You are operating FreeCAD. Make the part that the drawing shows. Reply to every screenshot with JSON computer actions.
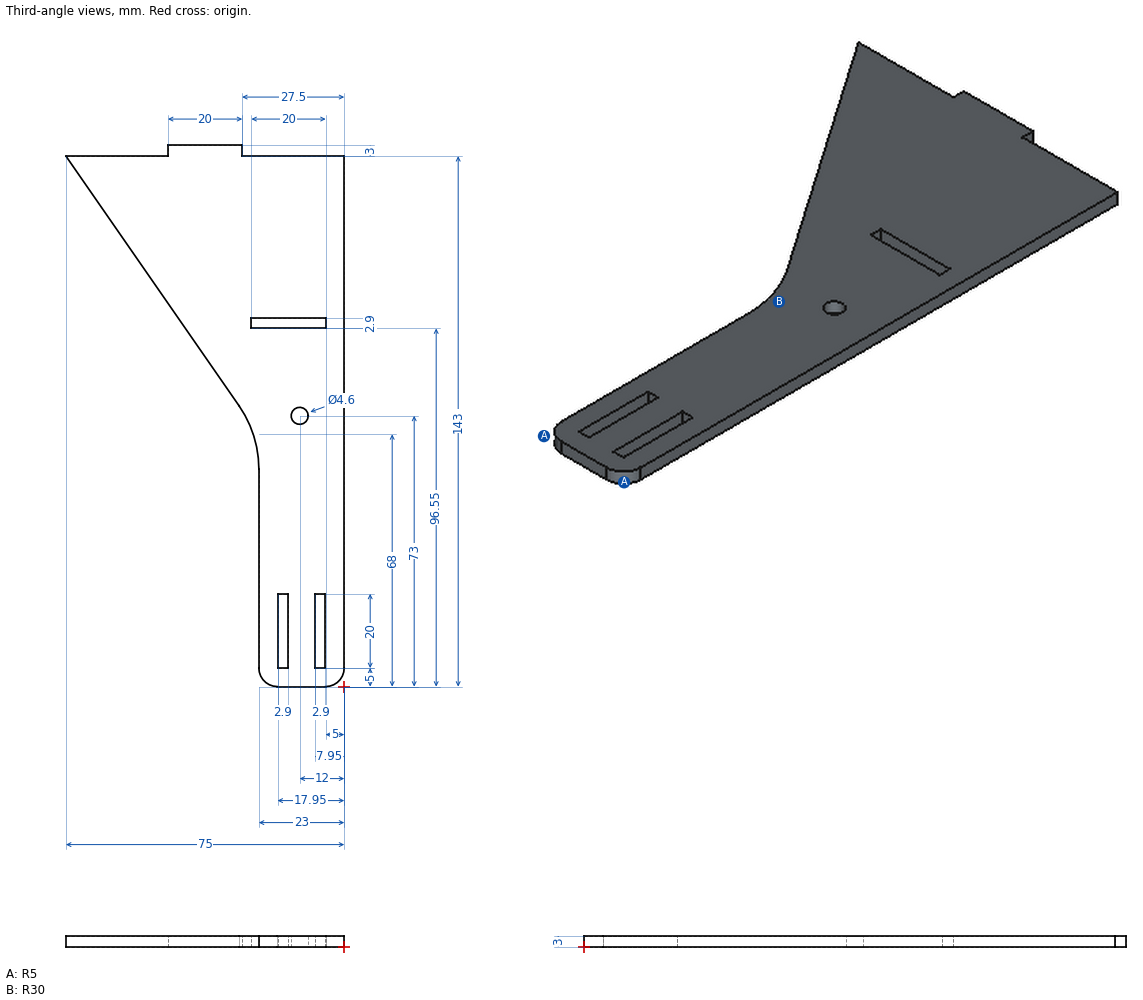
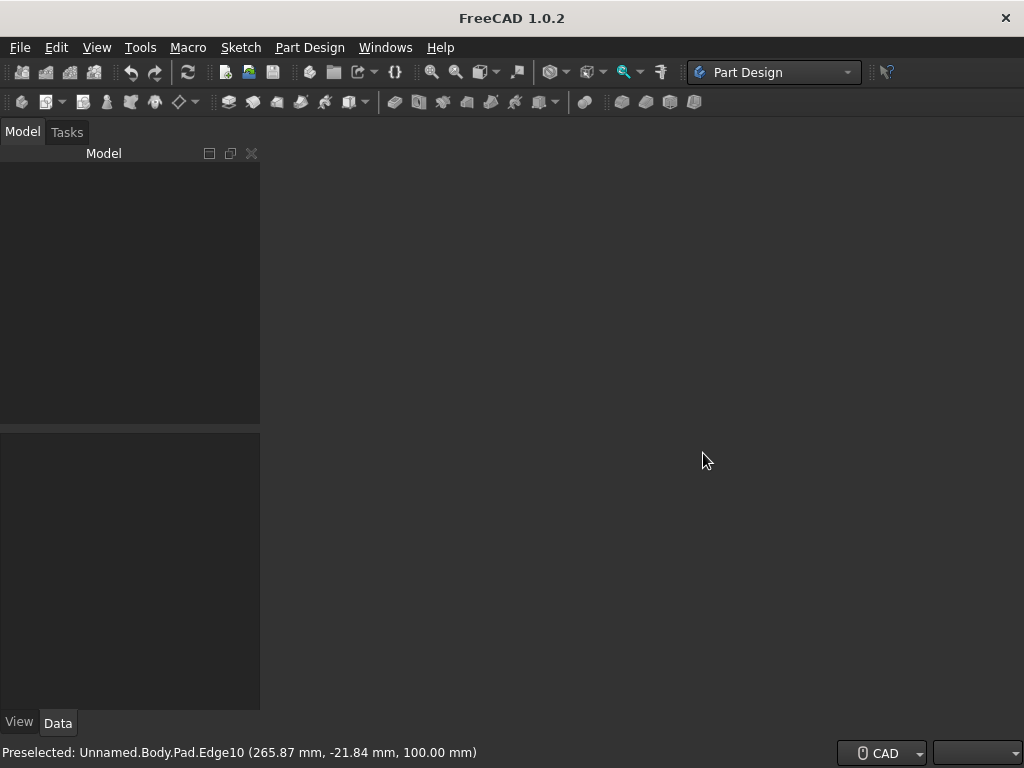
{"action": "left_click", "coordinate": [226, 72]}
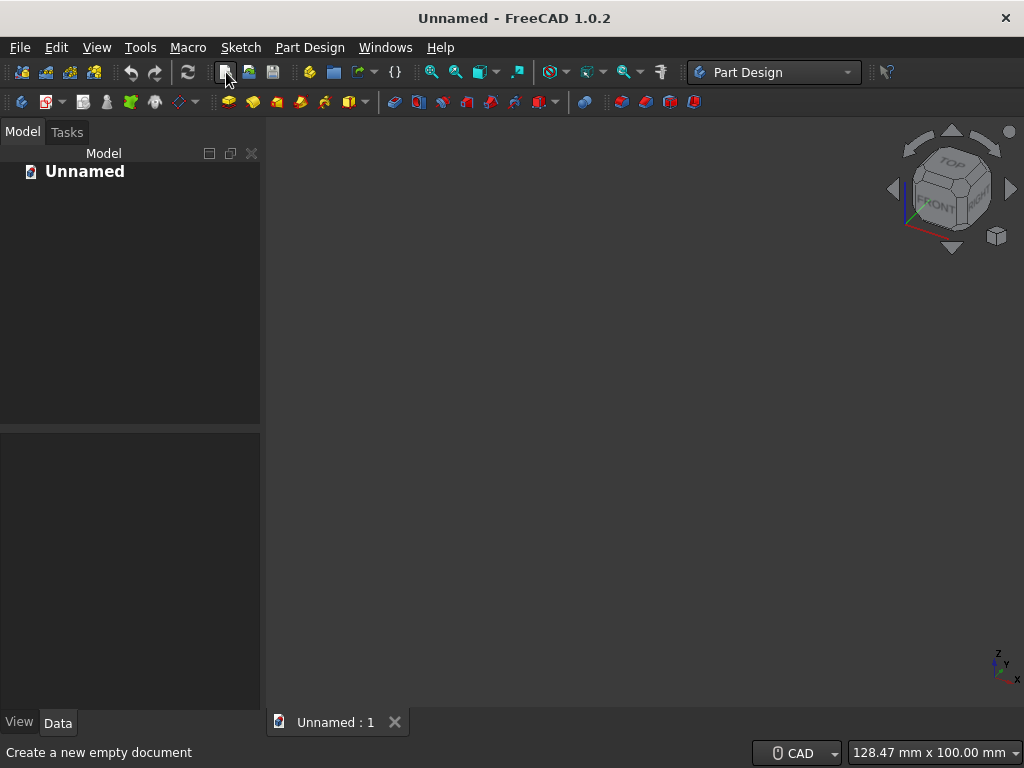
{"action": "left_click", "coordinate": [46, 102]}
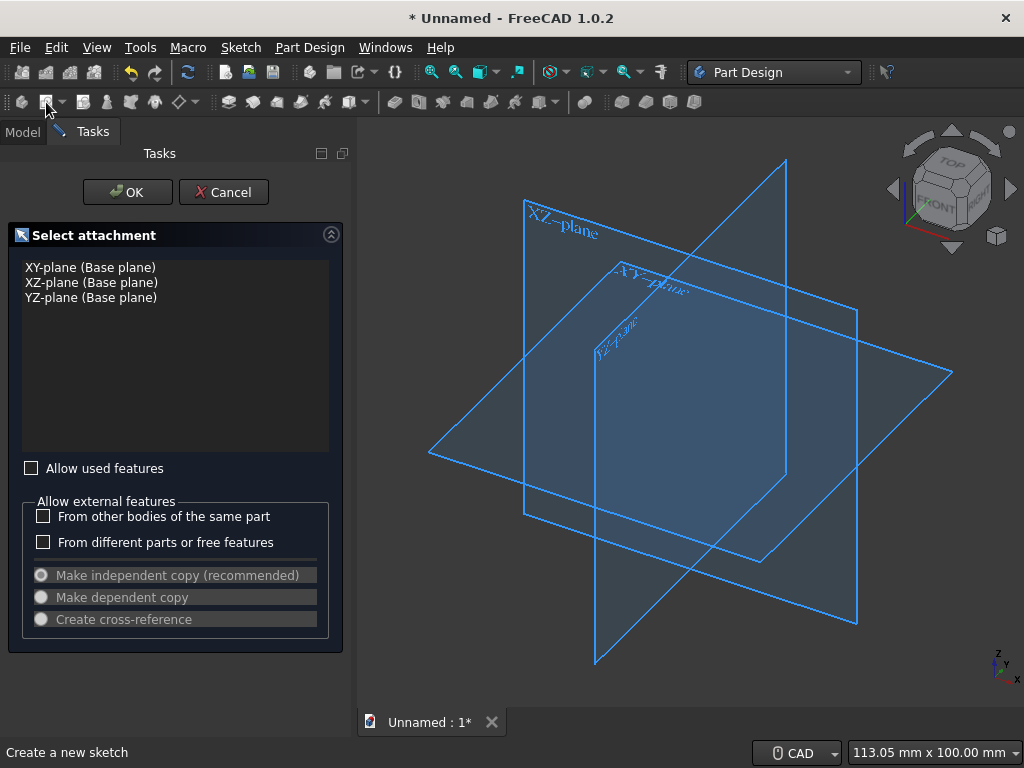
{"action": "left_click", "coordinate": [82, 268]}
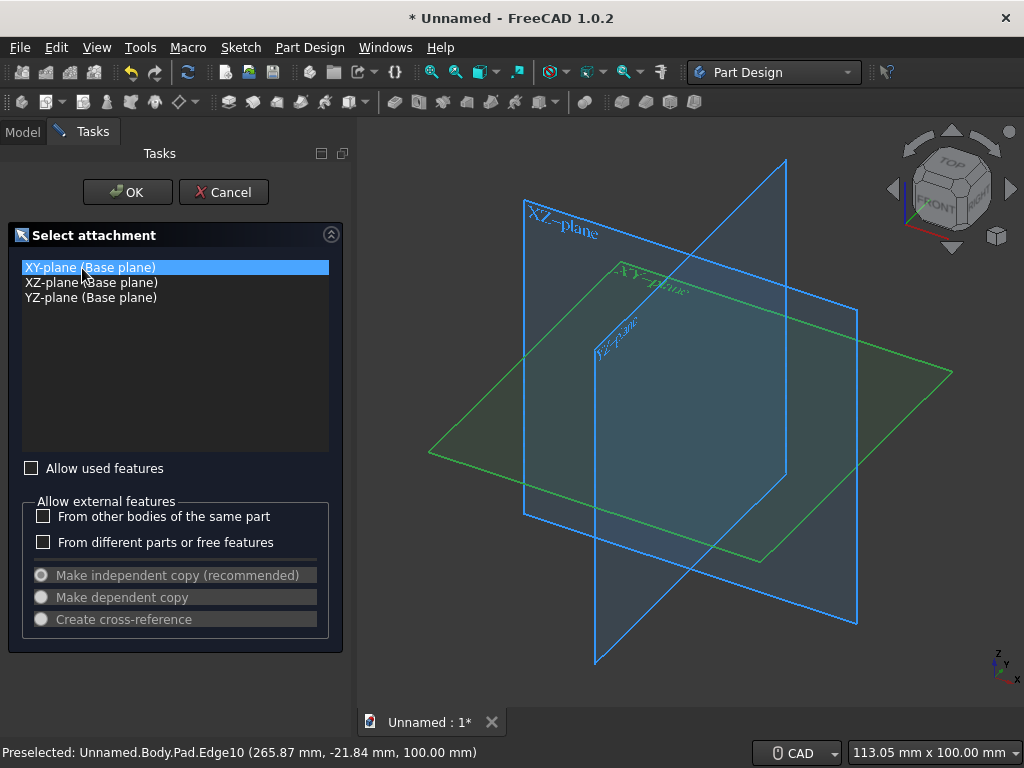
{"action": "left_click", "coordinate": [128, 192]}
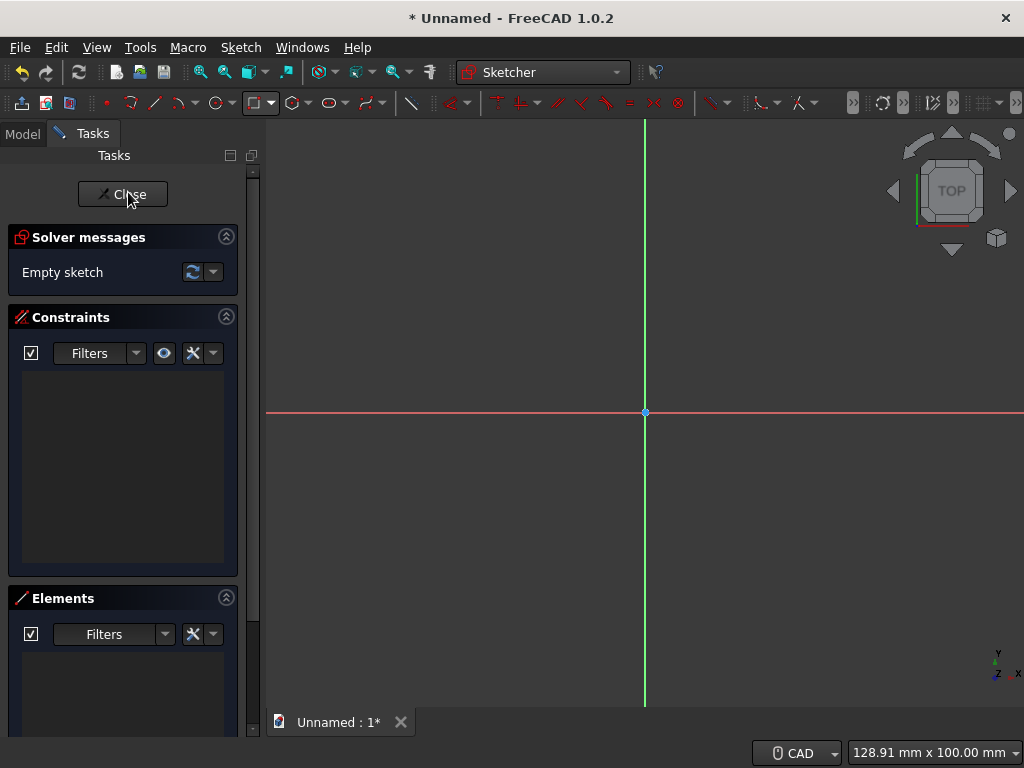
{"action": "scroll", "coordinate": [701, 679], "scroll_direction": "down", "scroll_amount": 4}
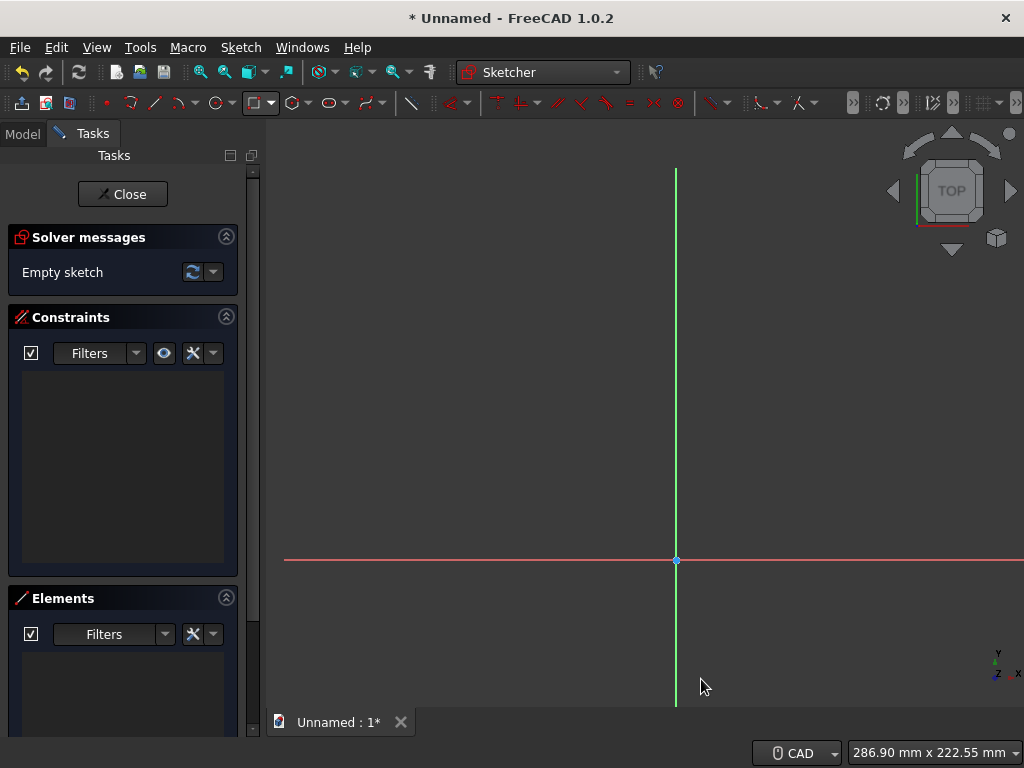
{"action": "left_click", "coordinate": [132, 104]}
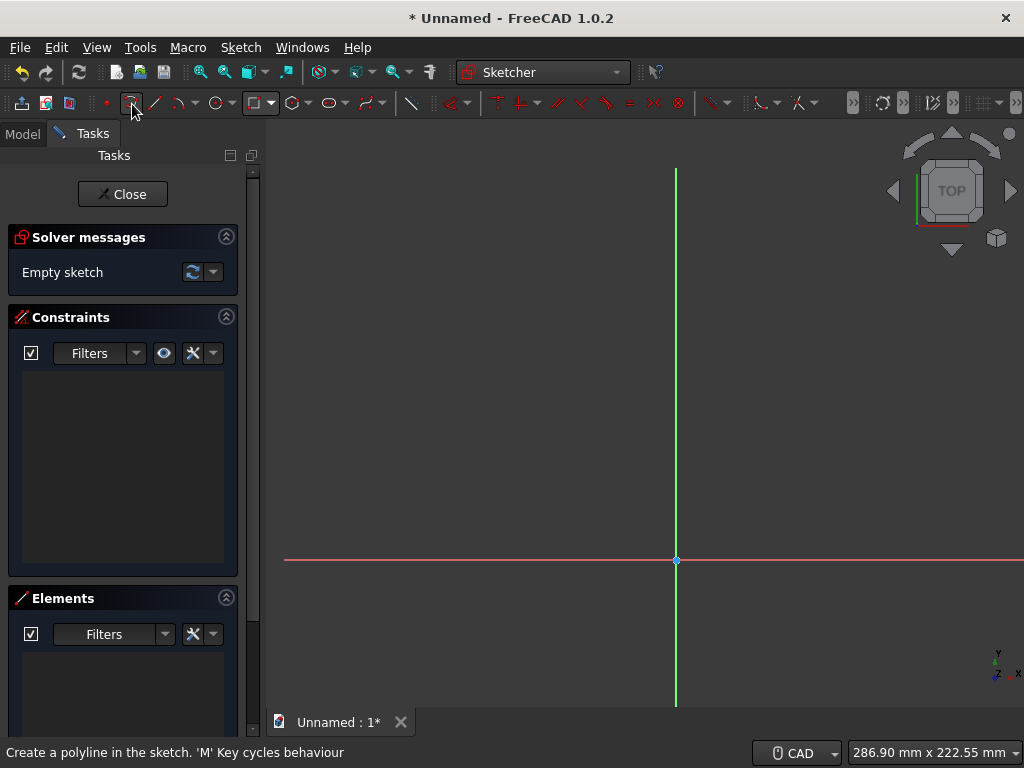
{"action": "left_click", "coordinate": [676, 560]}
{"action": "left_click", "coordinate": [667, 182]}
{"action": "left_click", "coordinate": [603, 182]}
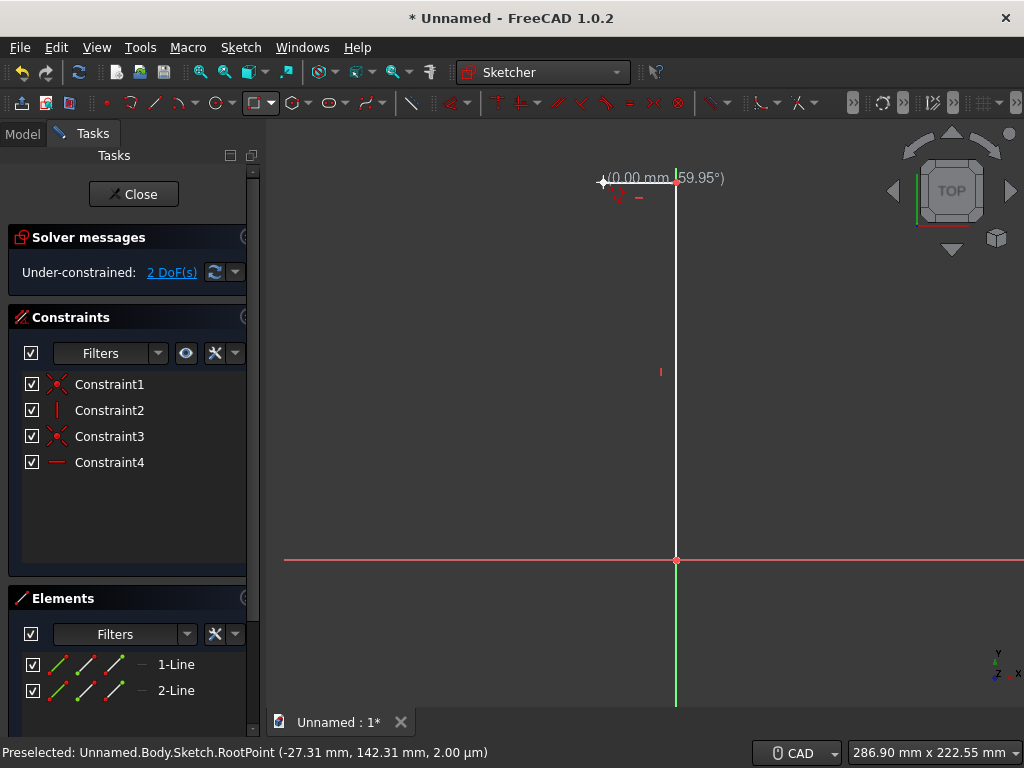
{"action": "scroll", "coordinate": [603, 174], "scroll_direction": "up", "scroll_amount": 4}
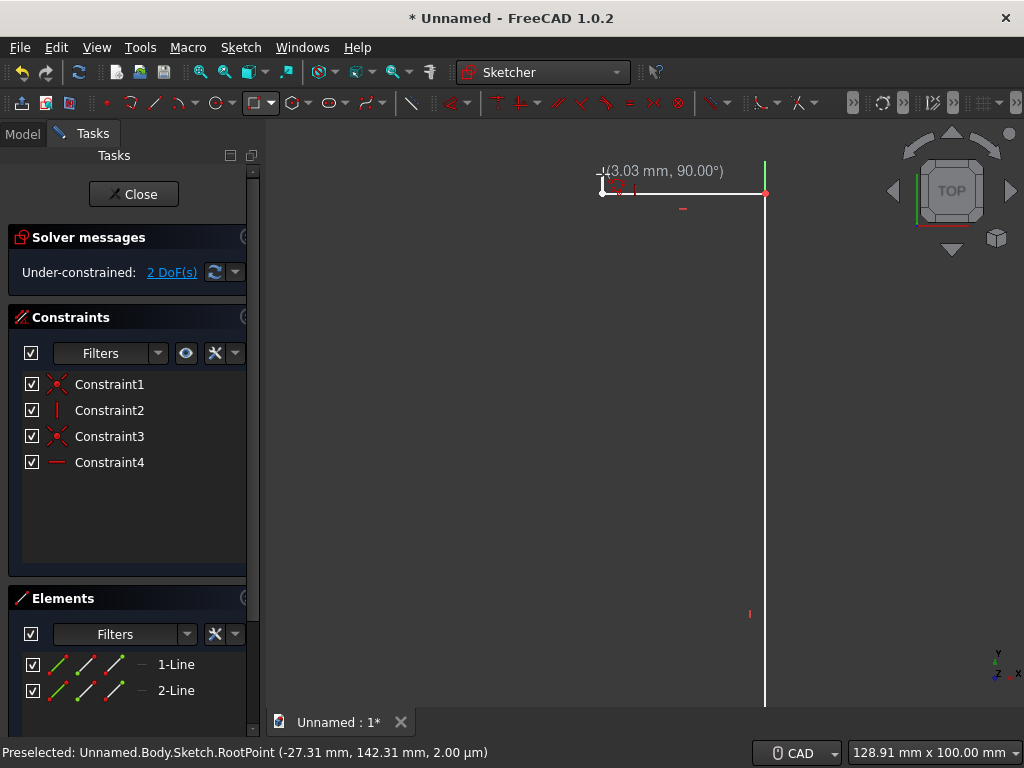
{"action": "left_click", "coordinate": [602, 174]}
{"action": "left_click", "coordinate": [486, 174]}
{"action": "left_click", "coordinate": [486, 192]}
{"action": "left_click", "coordinate": [324, 192]}
{"action": "left_click", "coordinate": [630, 633]}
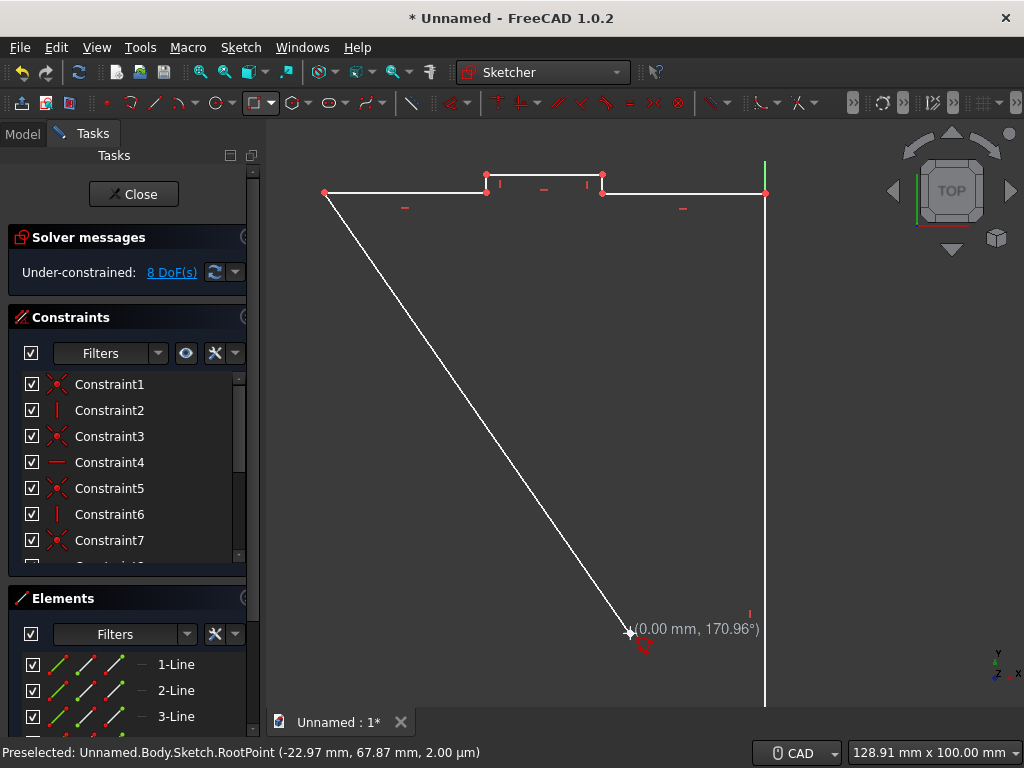
{"action": "scroll", "coordinate": [602, 257], "scroll_direction": "down", "scroll_amount": 4}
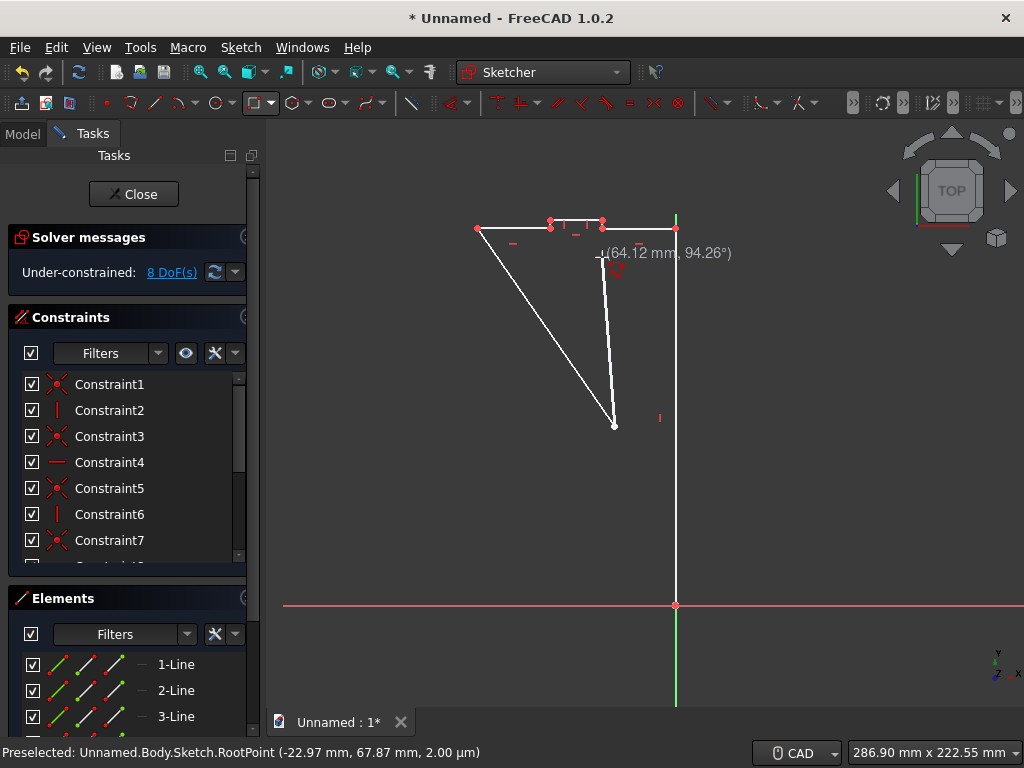
{"action": "left_click", "coordinate": [615, 597]}
{"action": "left_click", "coordinate": [676, 606]}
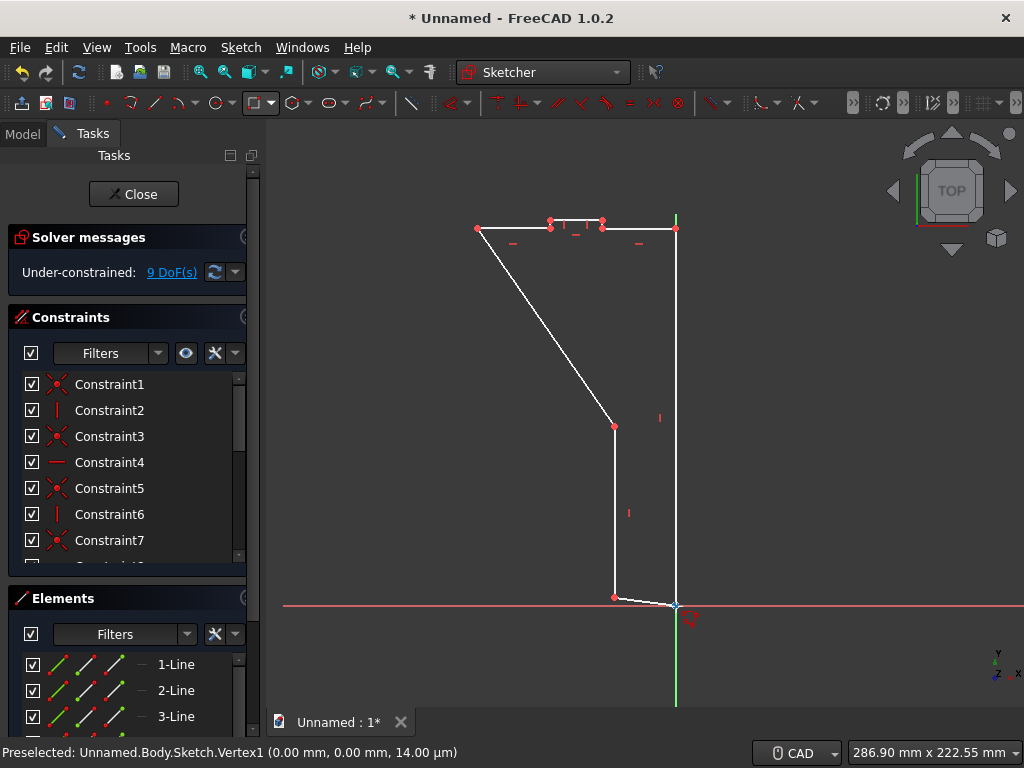
{"action": "key", "text": "g r"}